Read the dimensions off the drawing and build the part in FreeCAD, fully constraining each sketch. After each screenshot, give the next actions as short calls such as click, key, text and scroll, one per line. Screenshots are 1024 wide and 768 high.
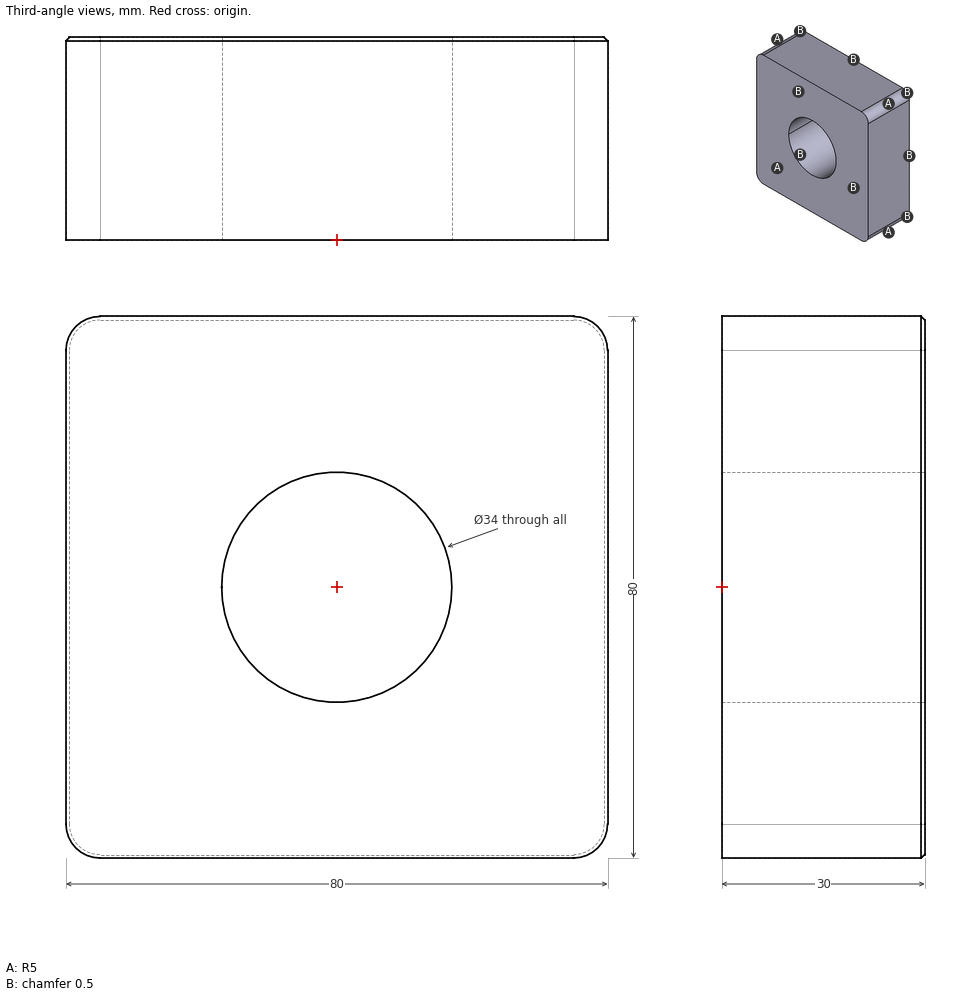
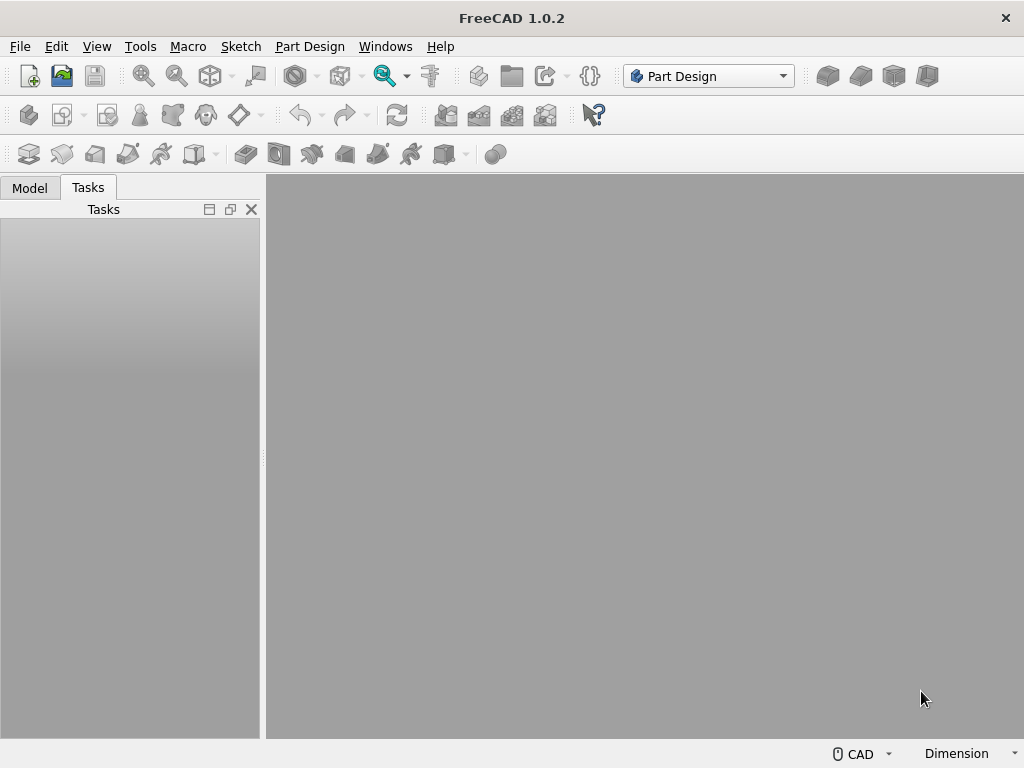
click(29, 76)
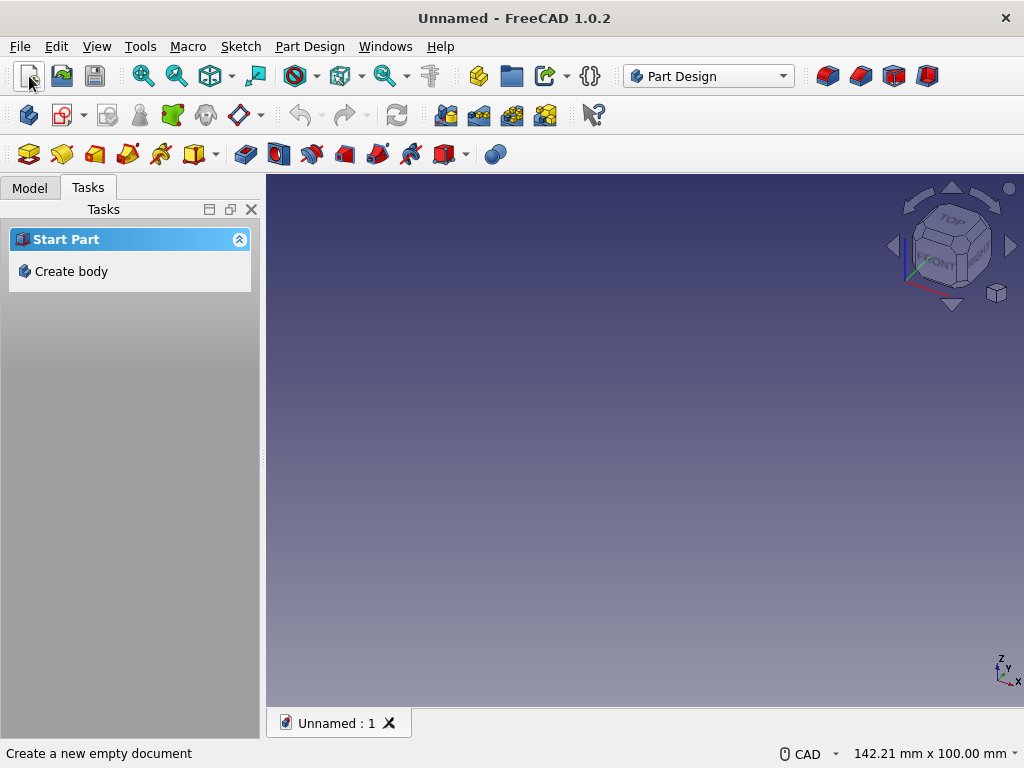
click(29, 116)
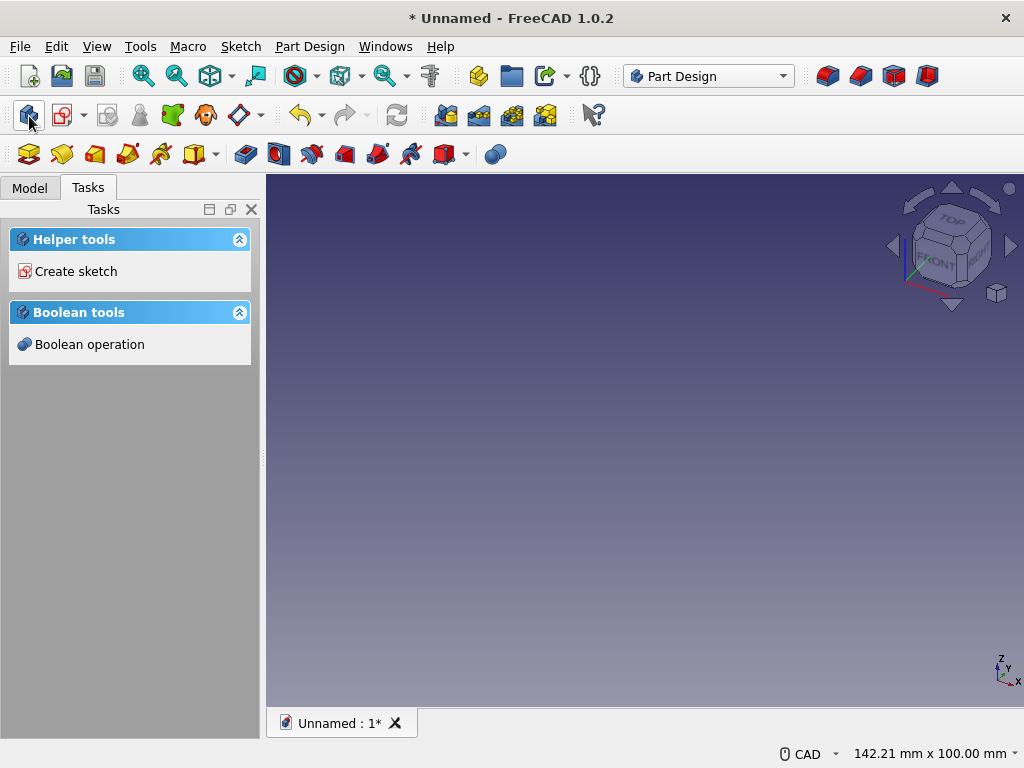
click(30, 188)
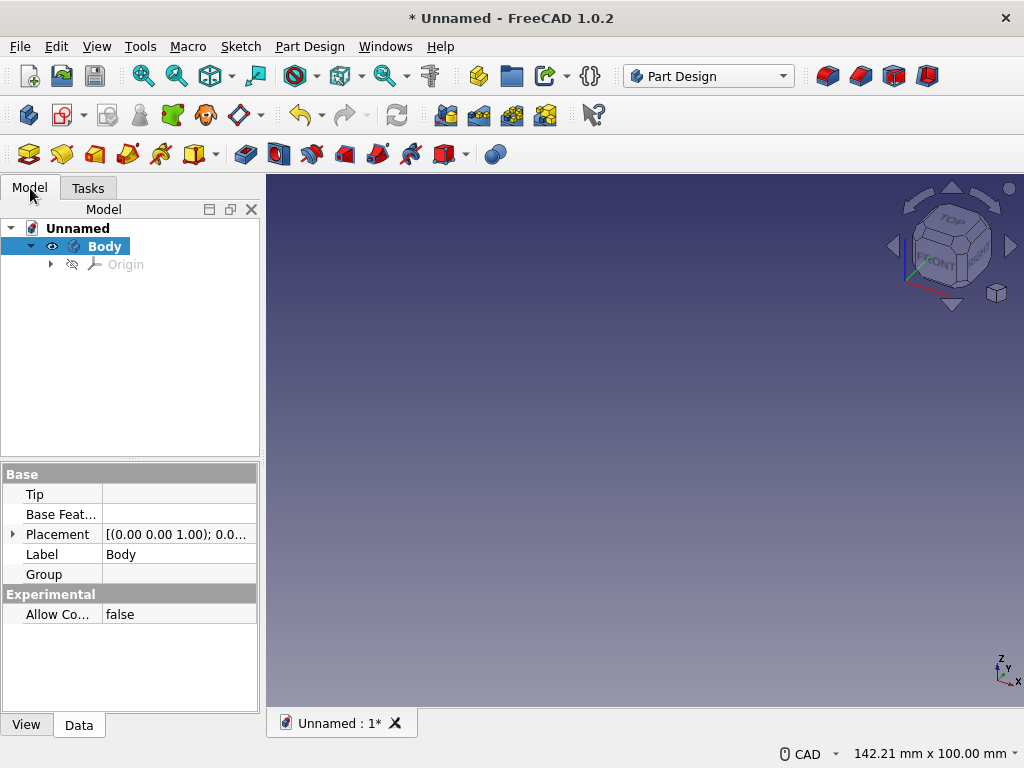
click(51, 264)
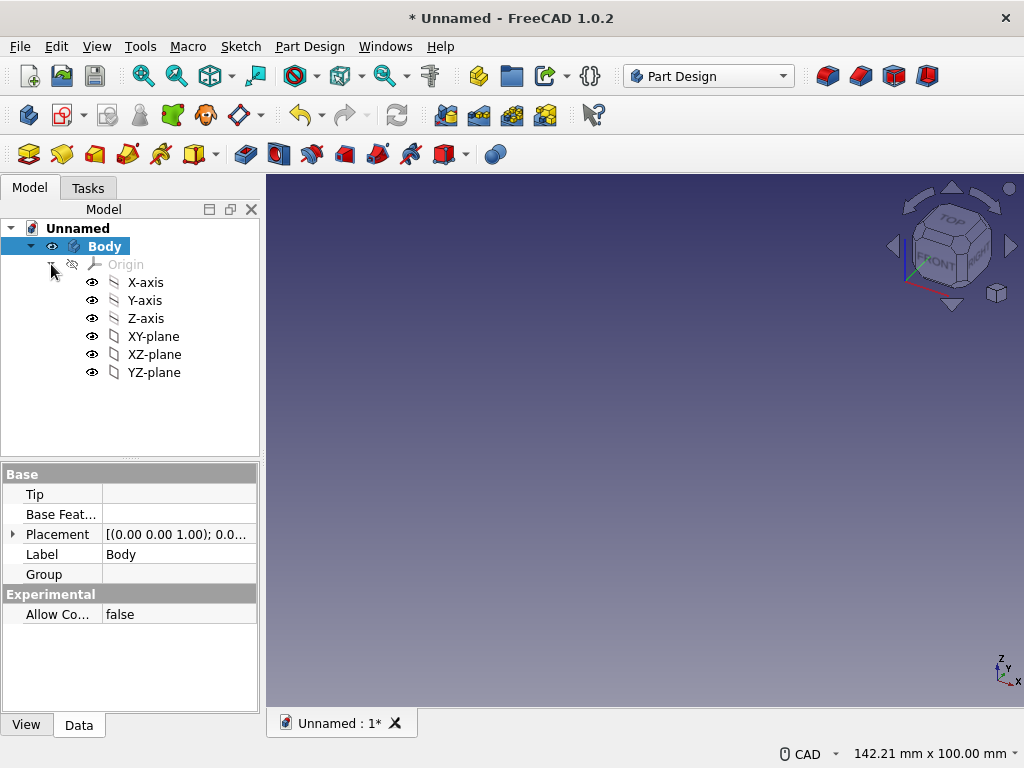
click(137, 354)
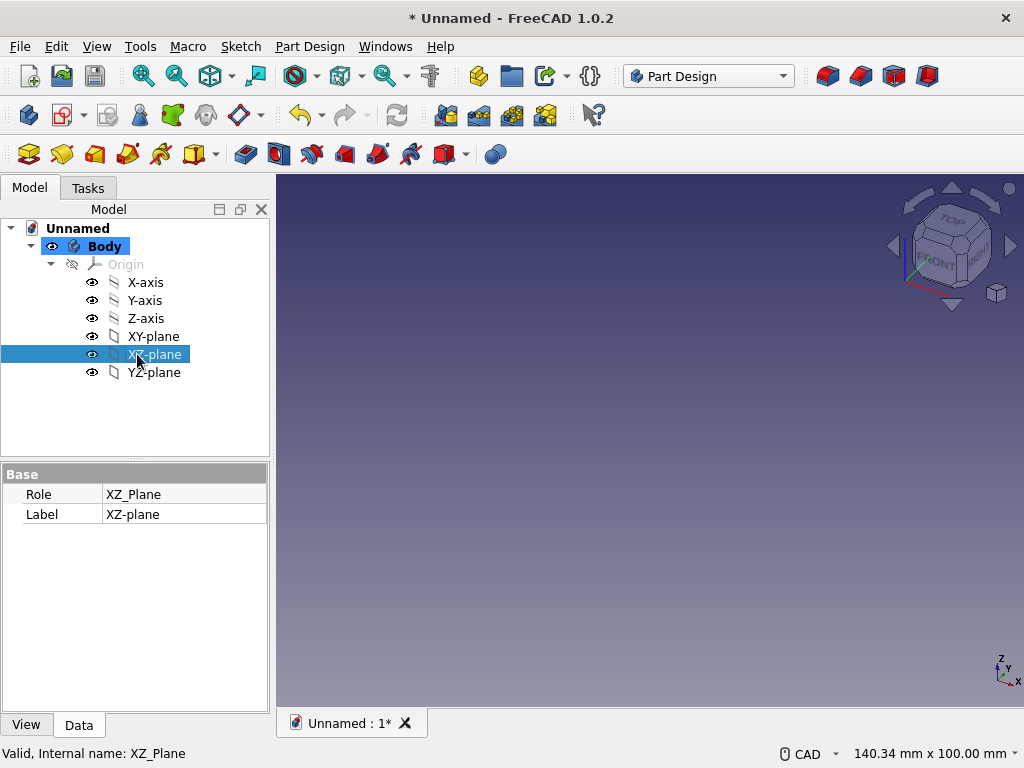
click(238, 116)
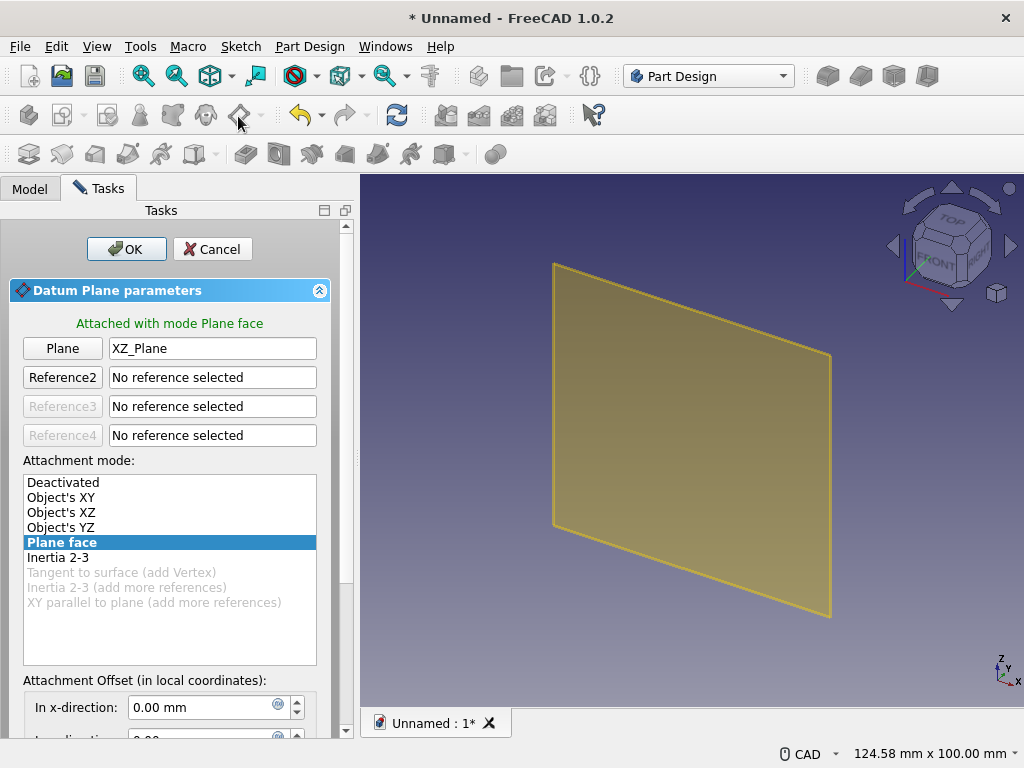
scroll(346, 479, down, 2)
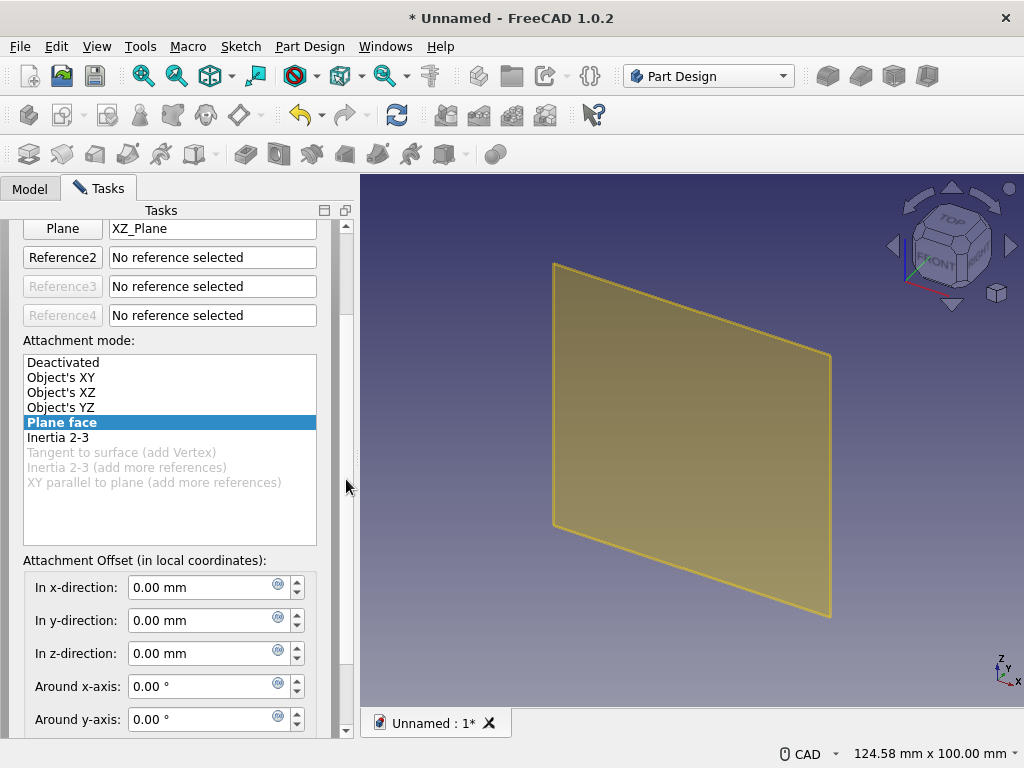
triple_click(210, 654)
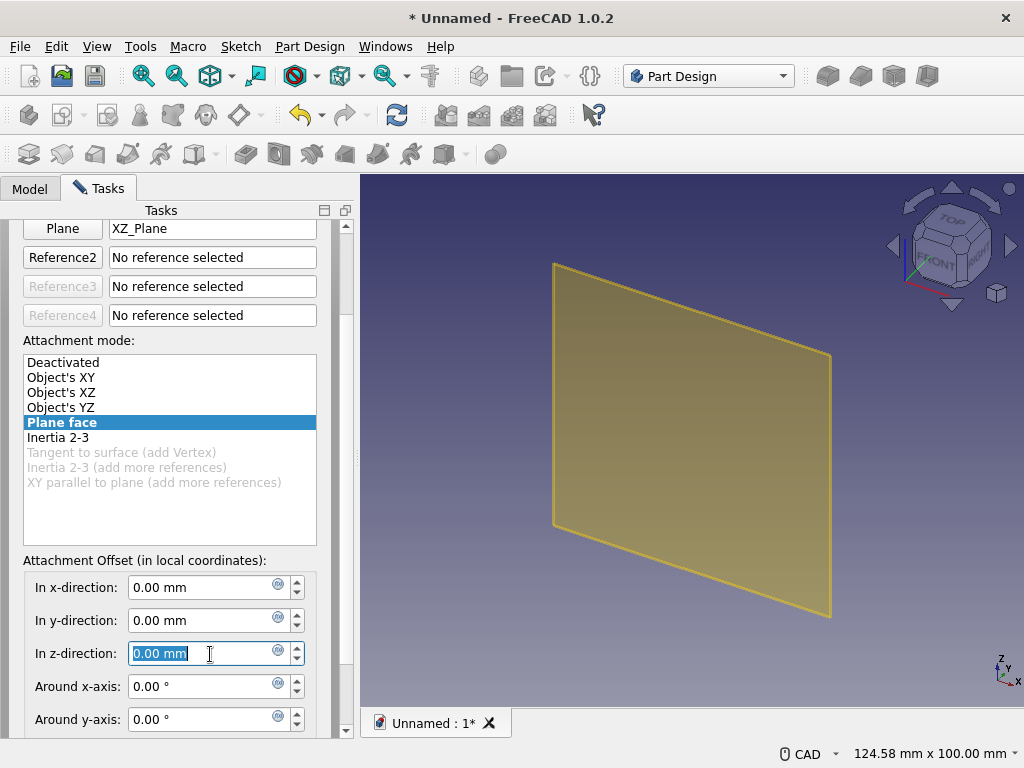
text(-30)
key(Tab)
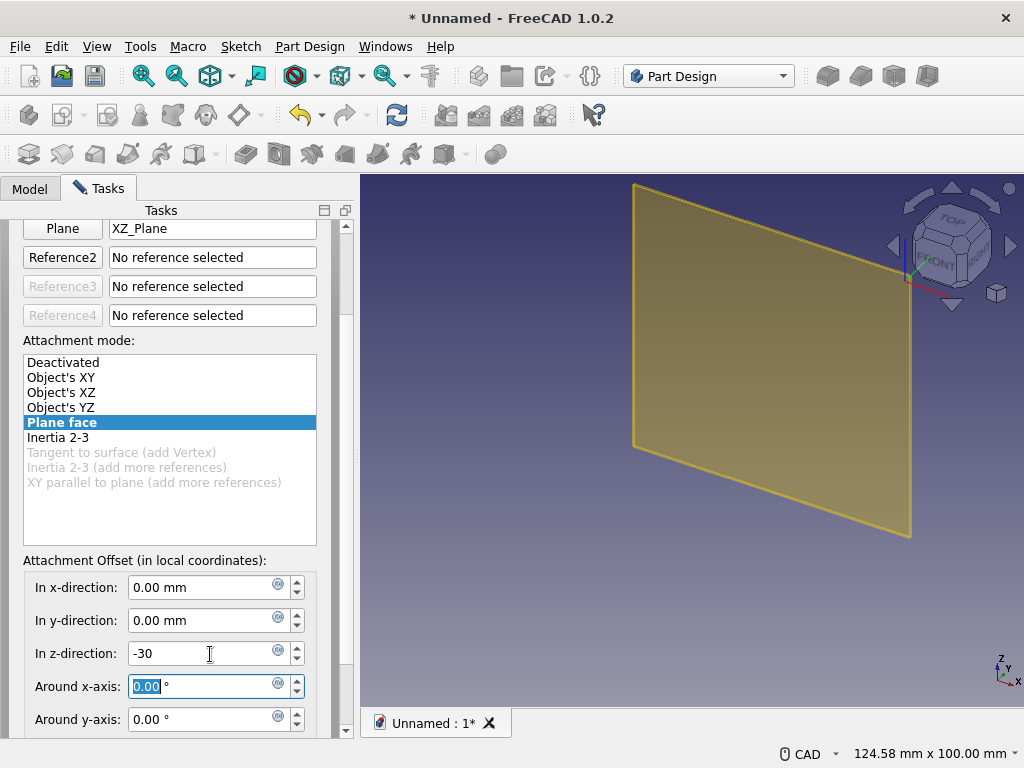
scroll(346, 479, up, 3)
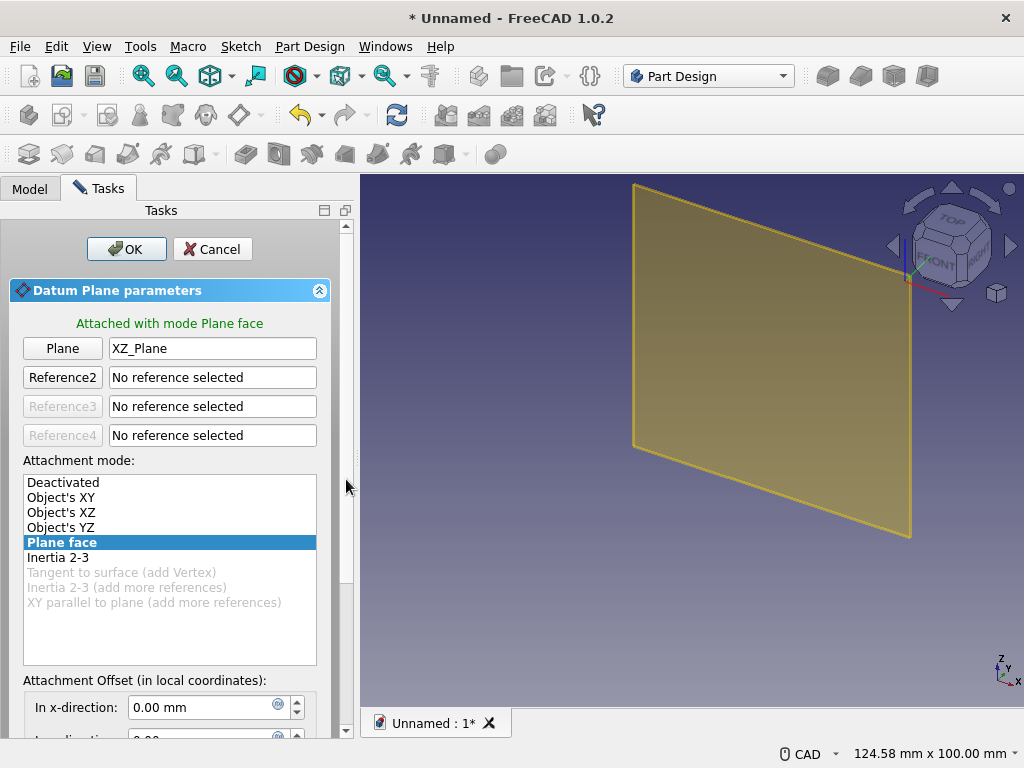
click(127, 249)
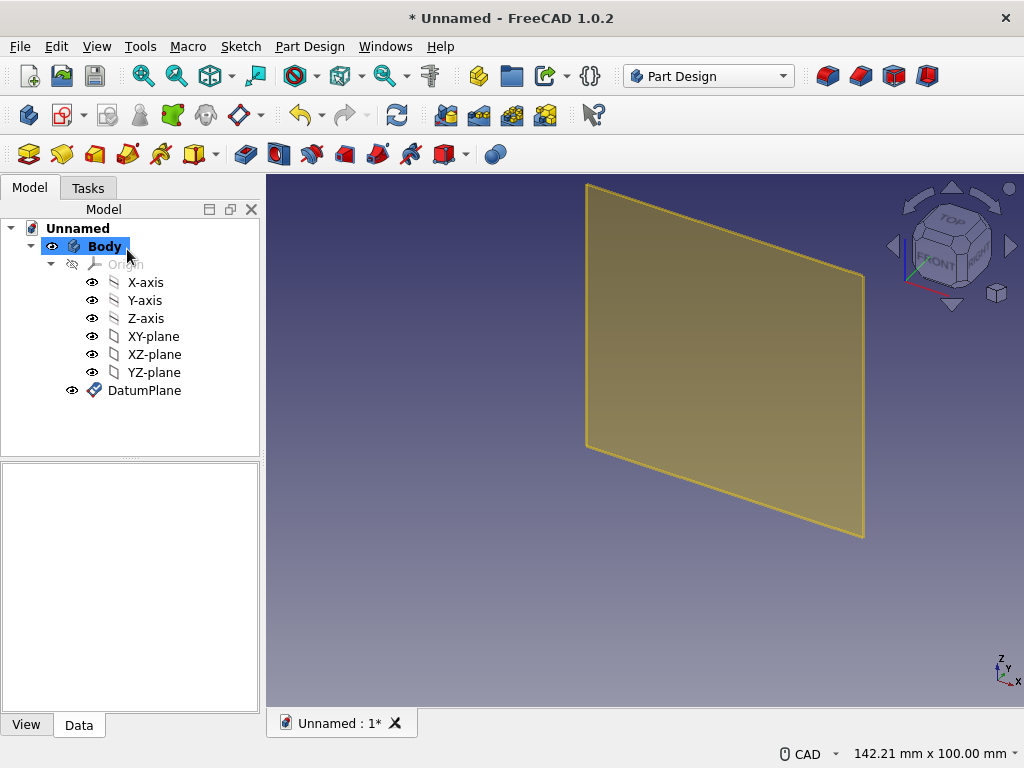
click(117, 390)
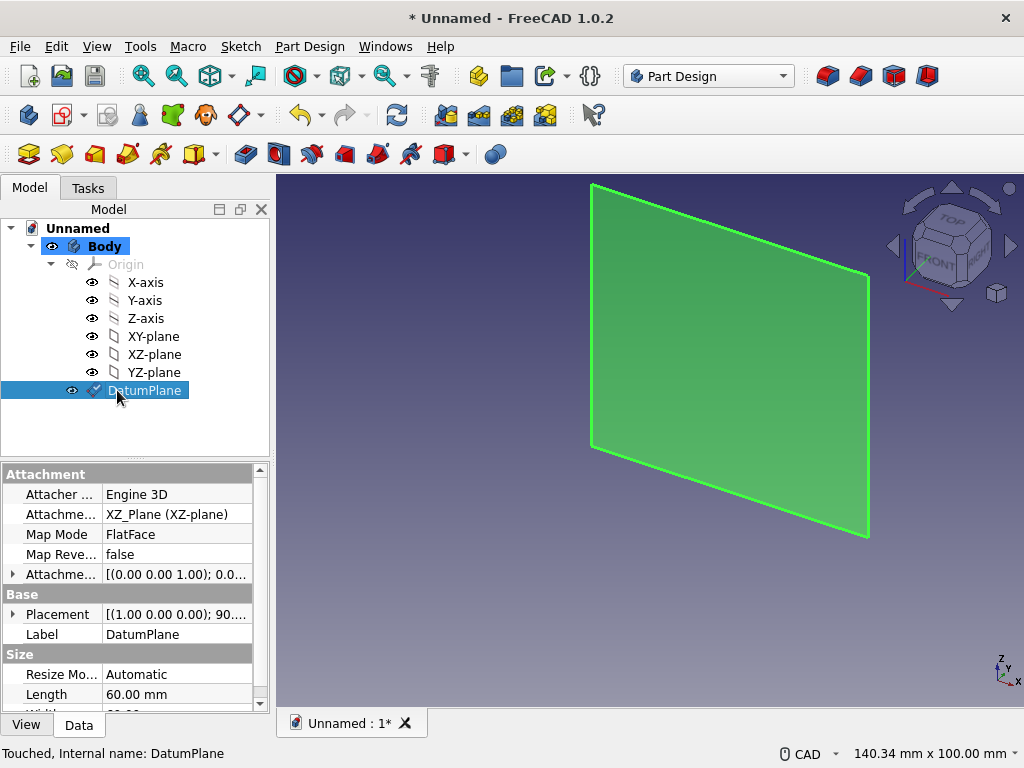
click(62, 116)